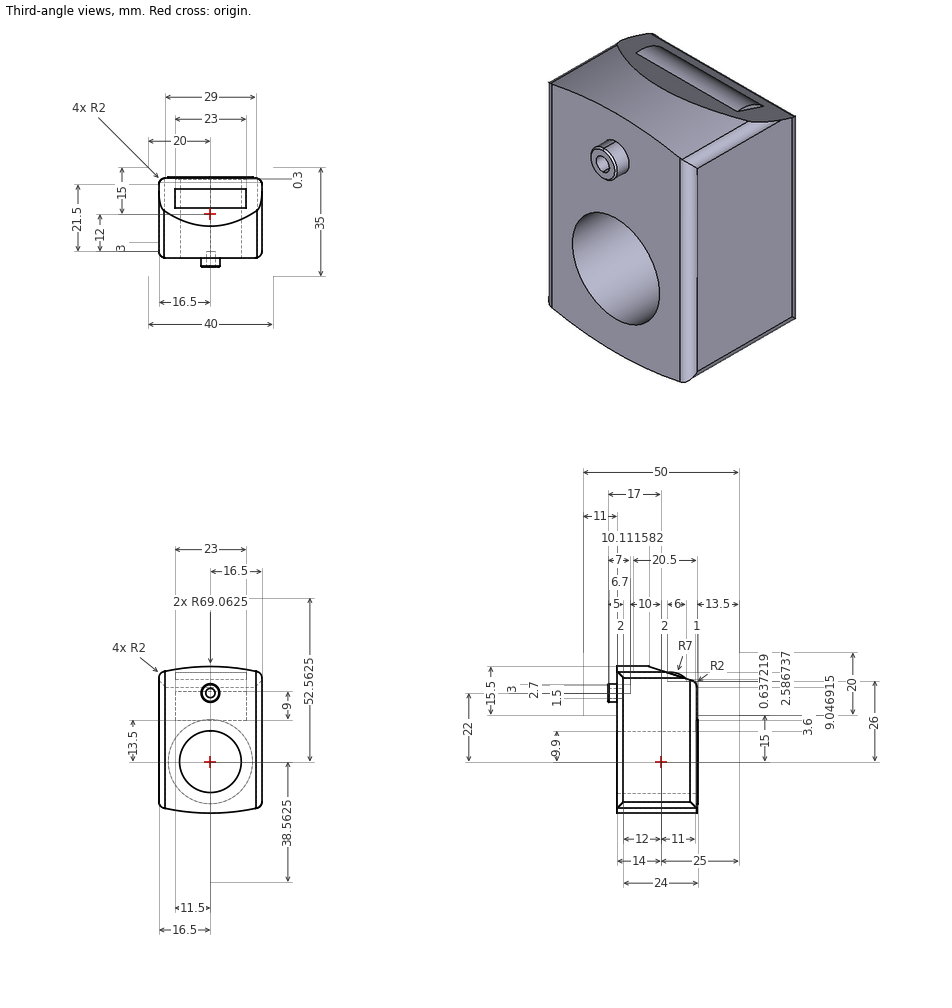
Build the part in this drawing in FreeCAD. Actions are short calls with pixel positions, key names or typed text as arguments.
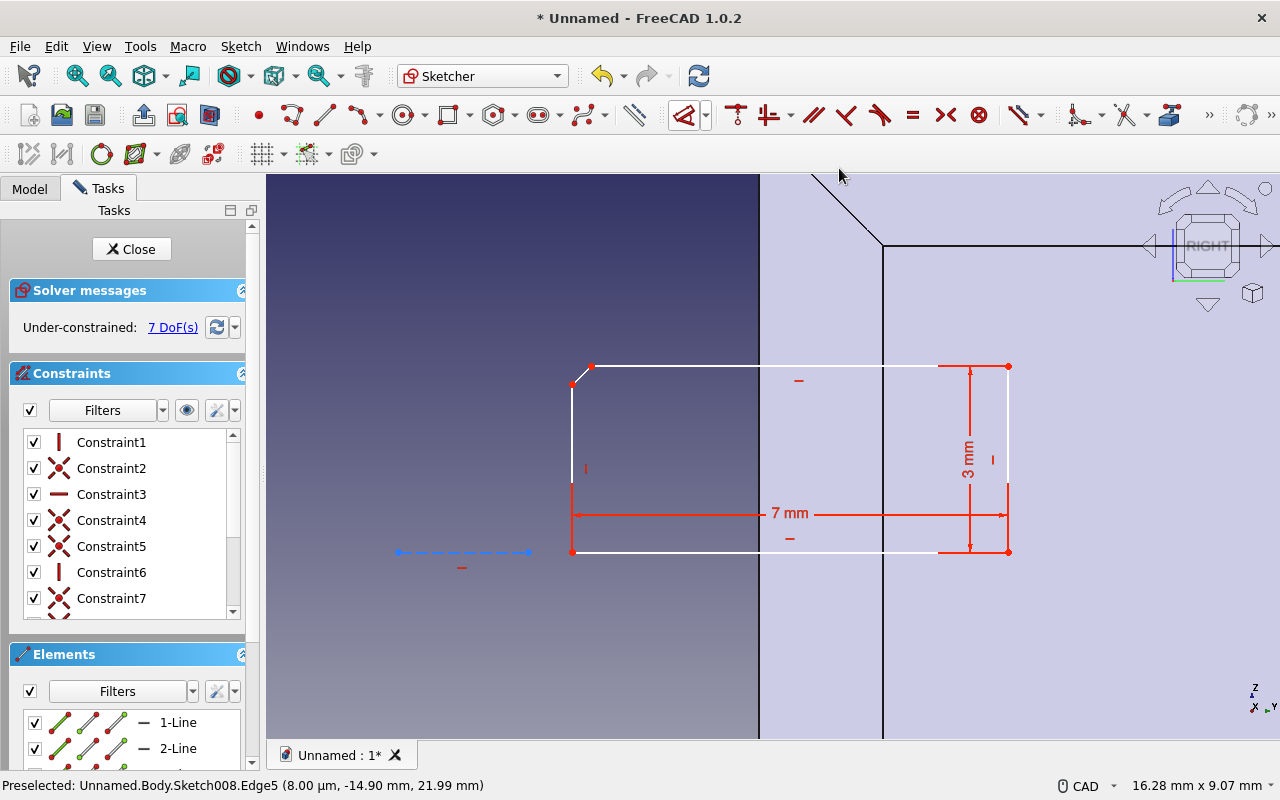
click(883, 366)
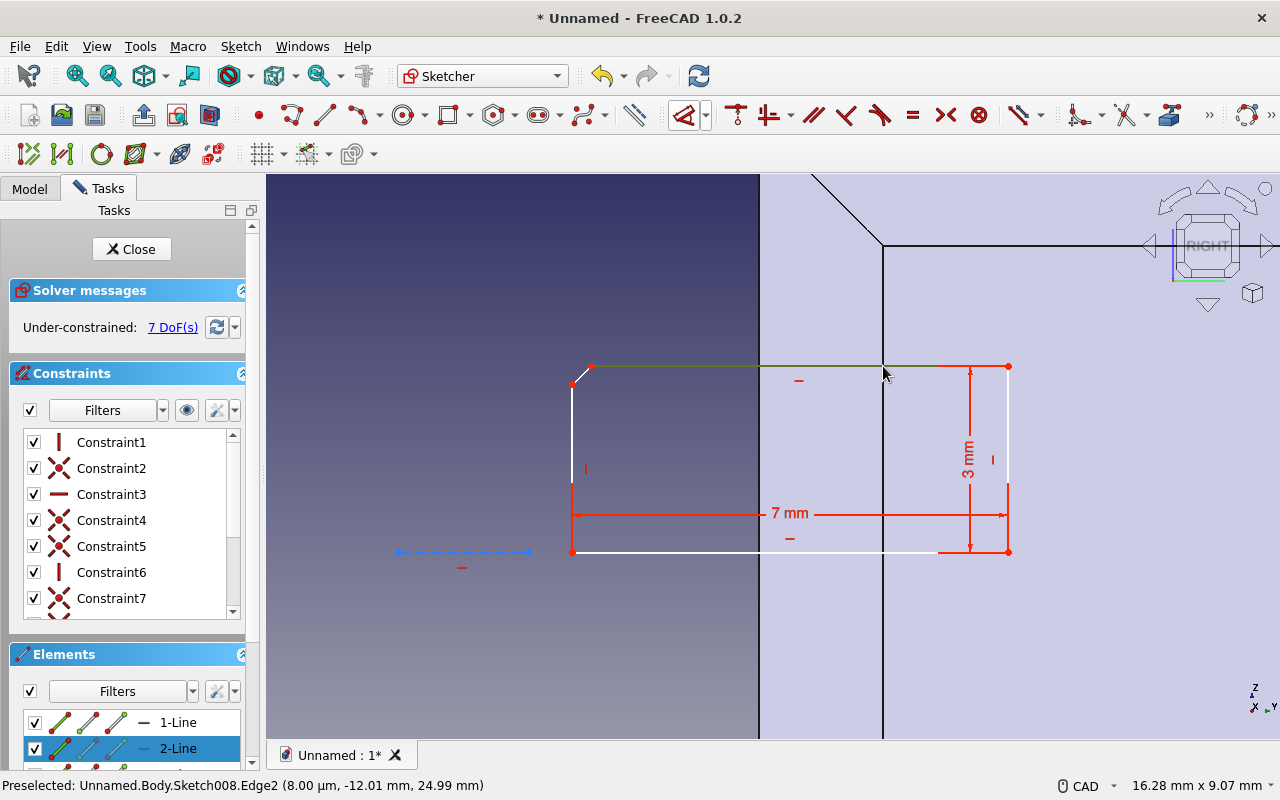
click(706, 116)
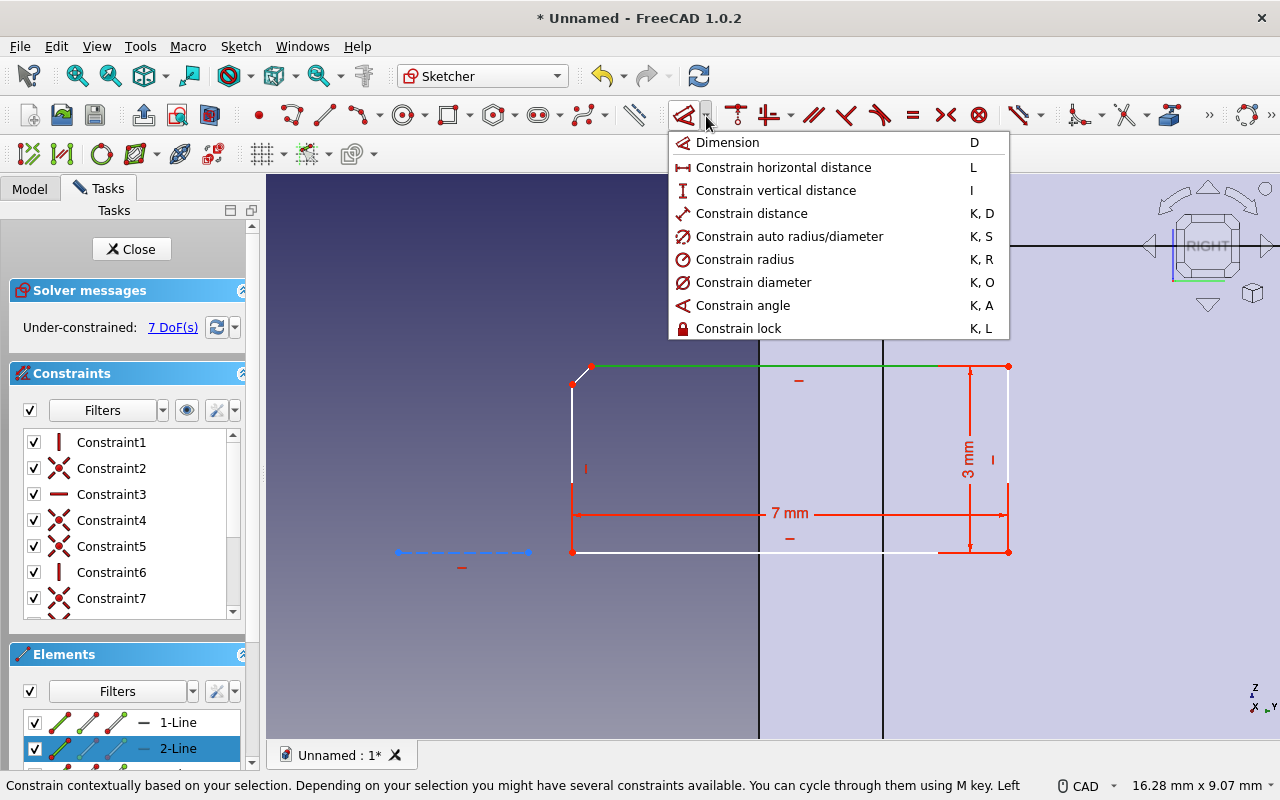
click(839, 168)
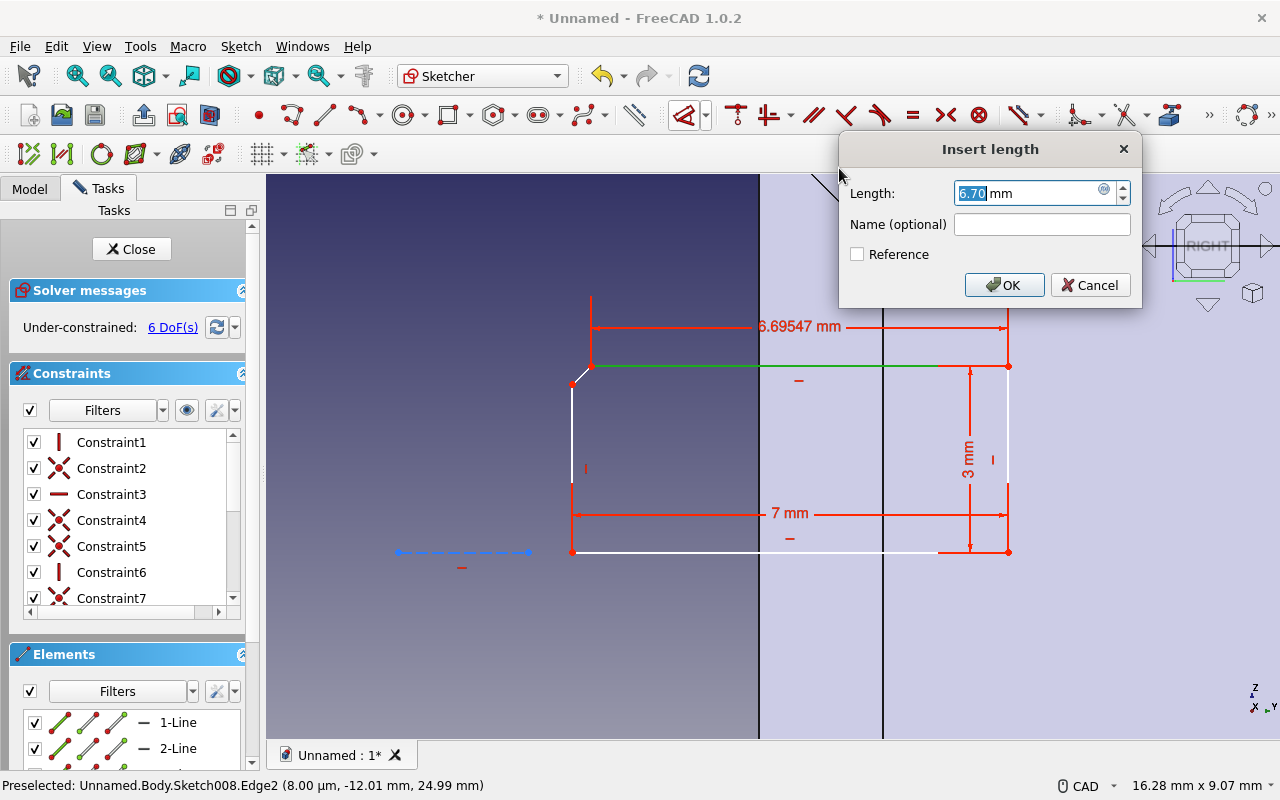
text(6.7)
key(Return)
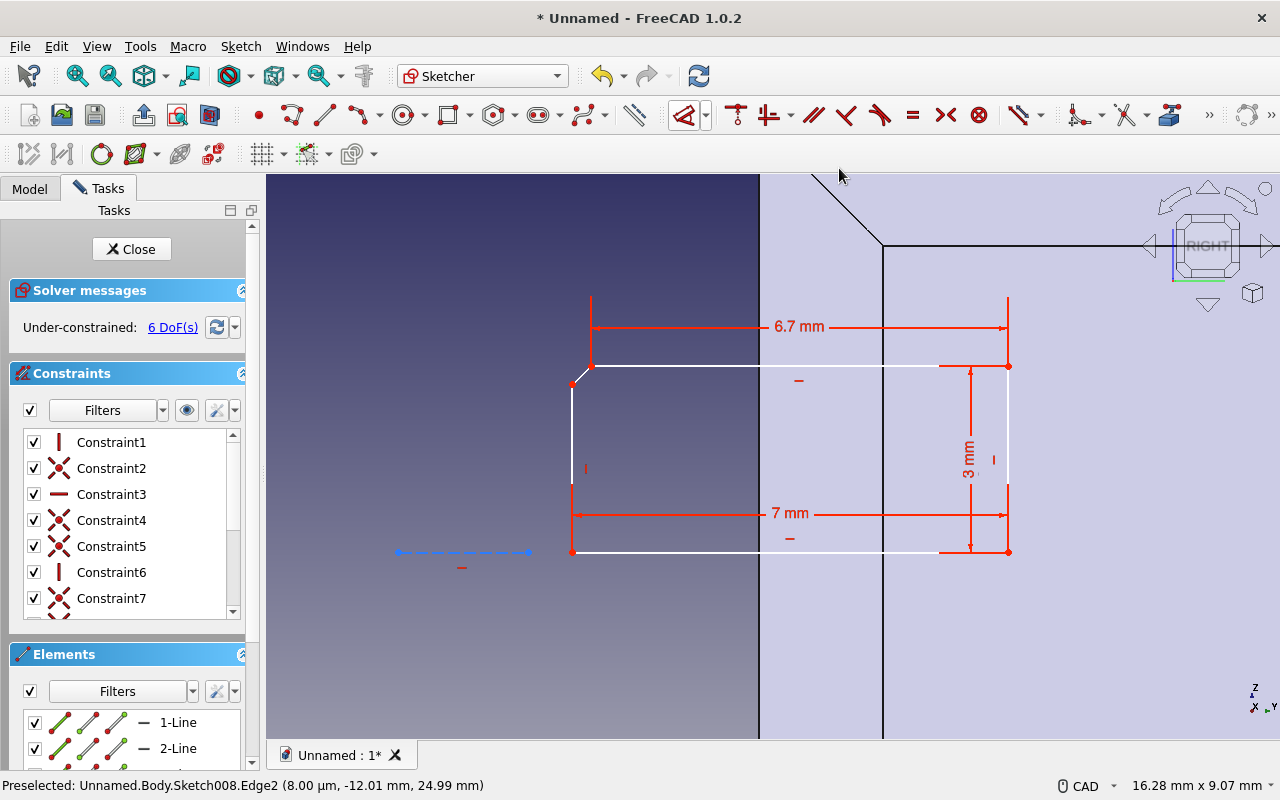
click(572, 435)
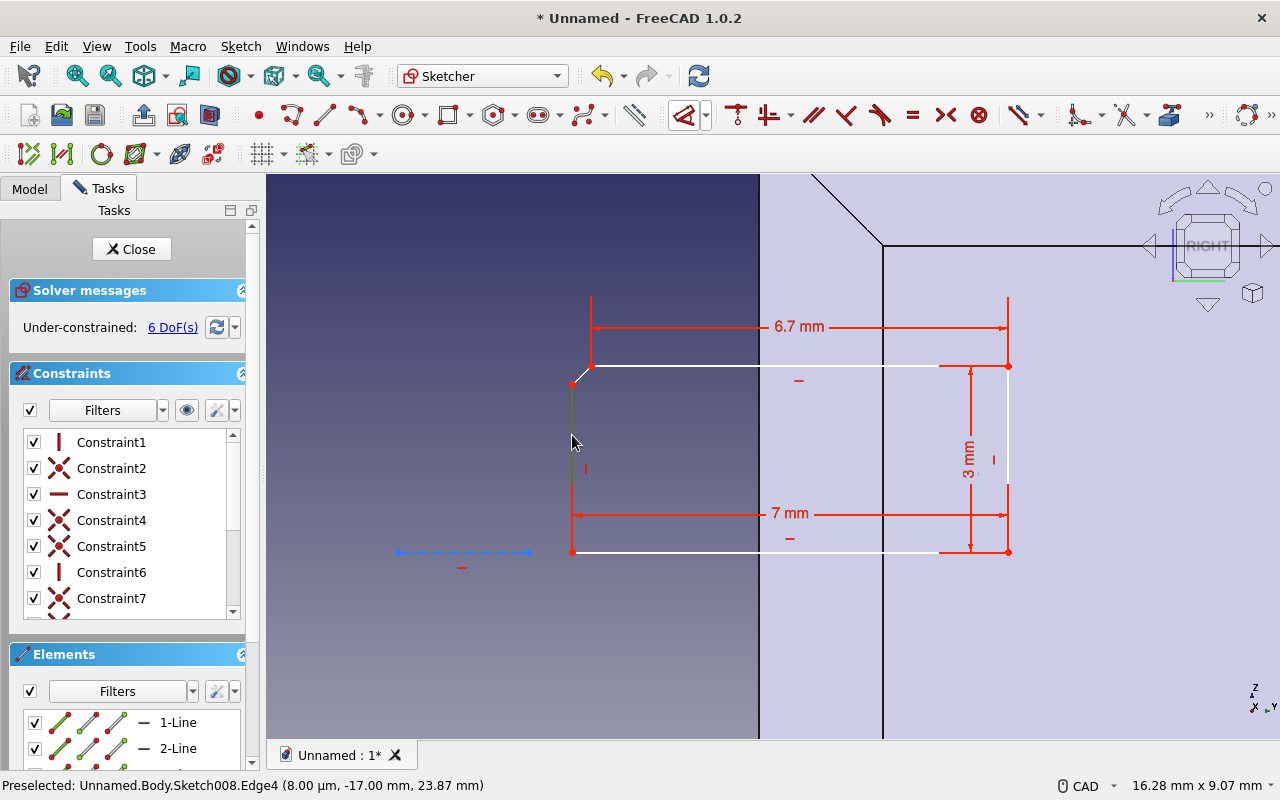
key(i)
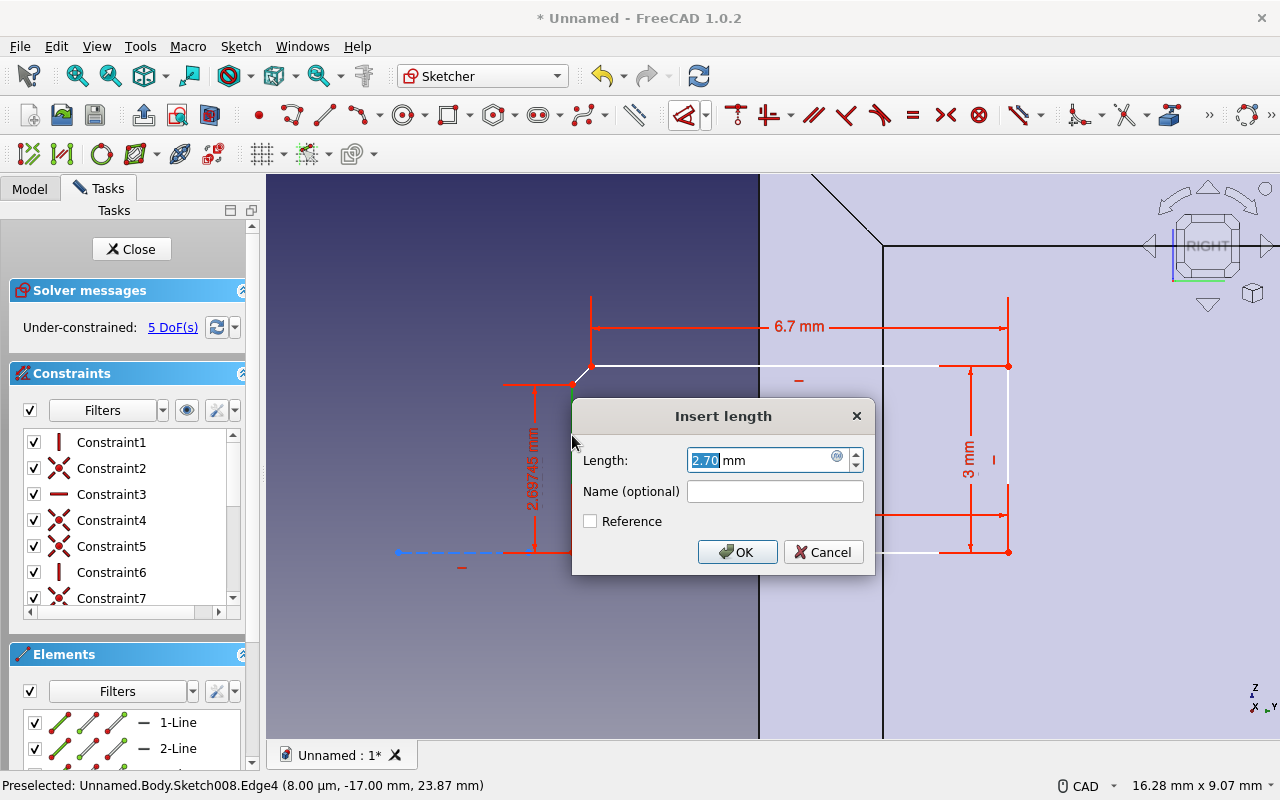
text(2.7)
key(Return)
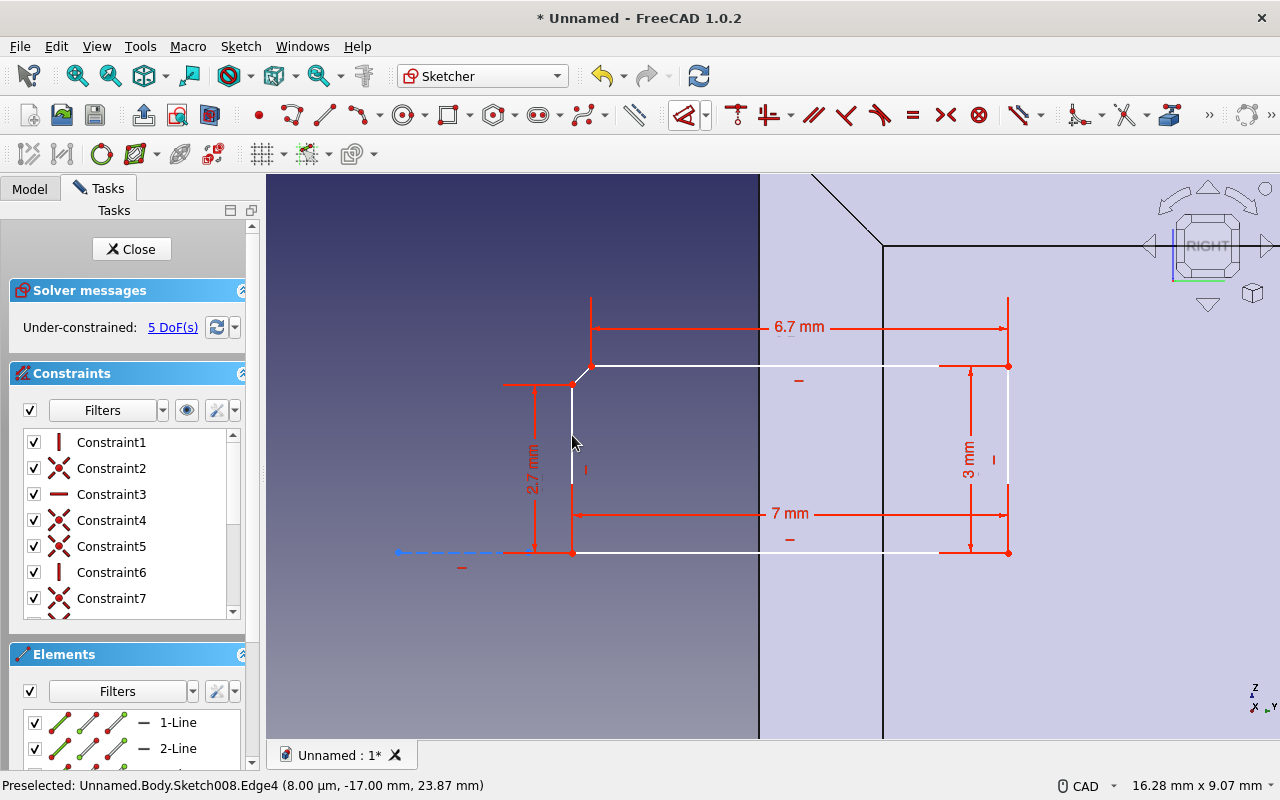
click(1008, 553)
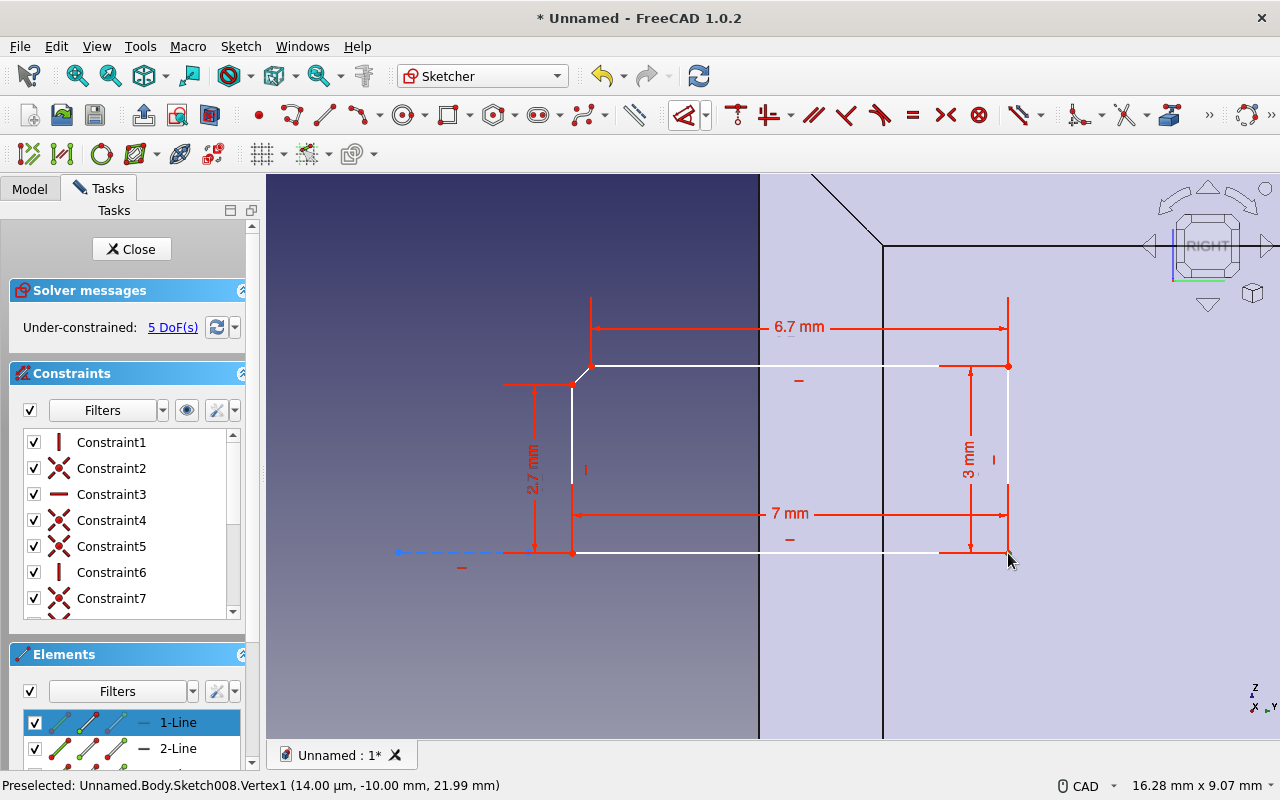
click(706, 116)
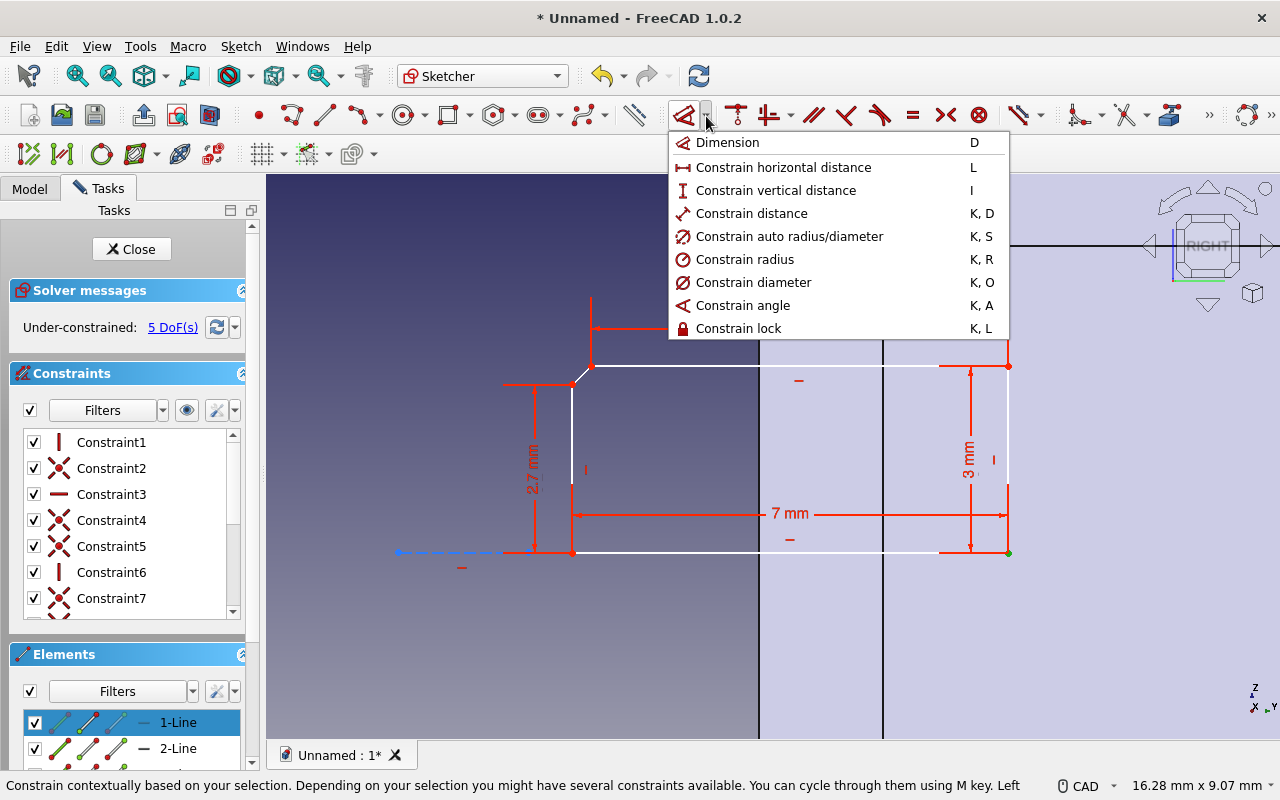
click(839, 168)